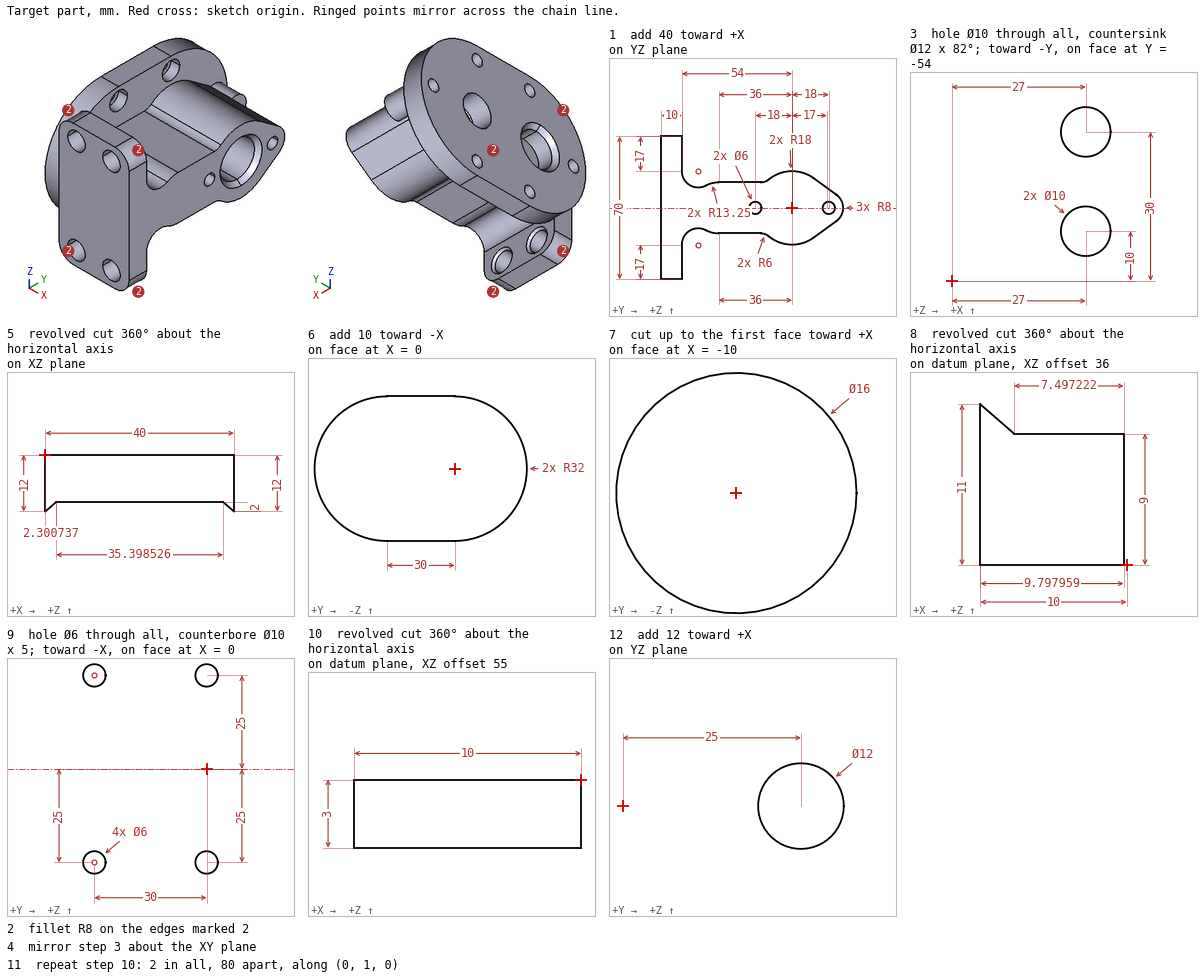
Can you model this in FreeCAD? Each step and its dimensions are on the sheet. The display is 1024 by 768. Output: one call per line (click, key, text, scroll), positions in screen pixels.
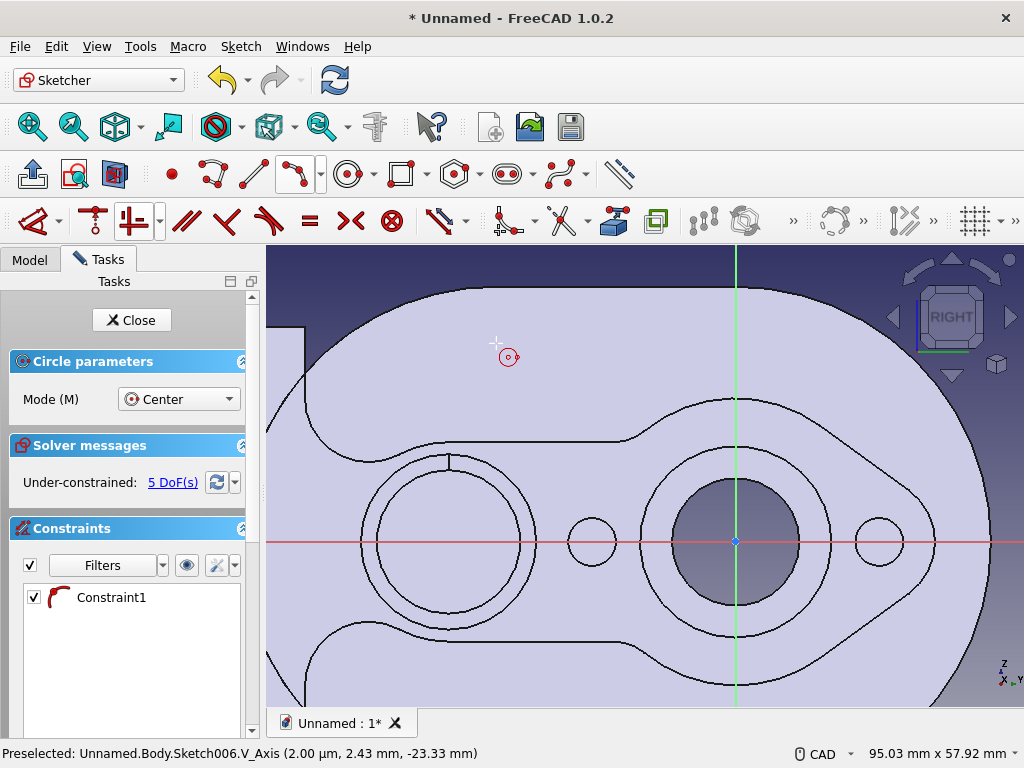
click(496, 343)
click(513, 326)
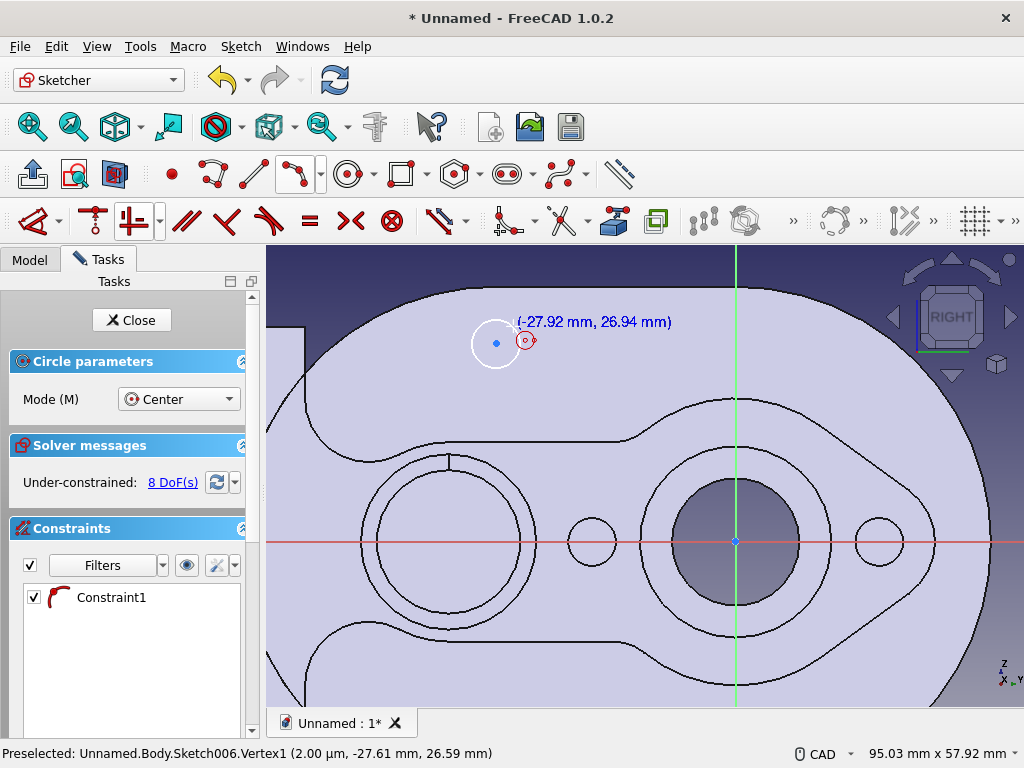
click(736, 343)
click(753, 326)
key(Escape)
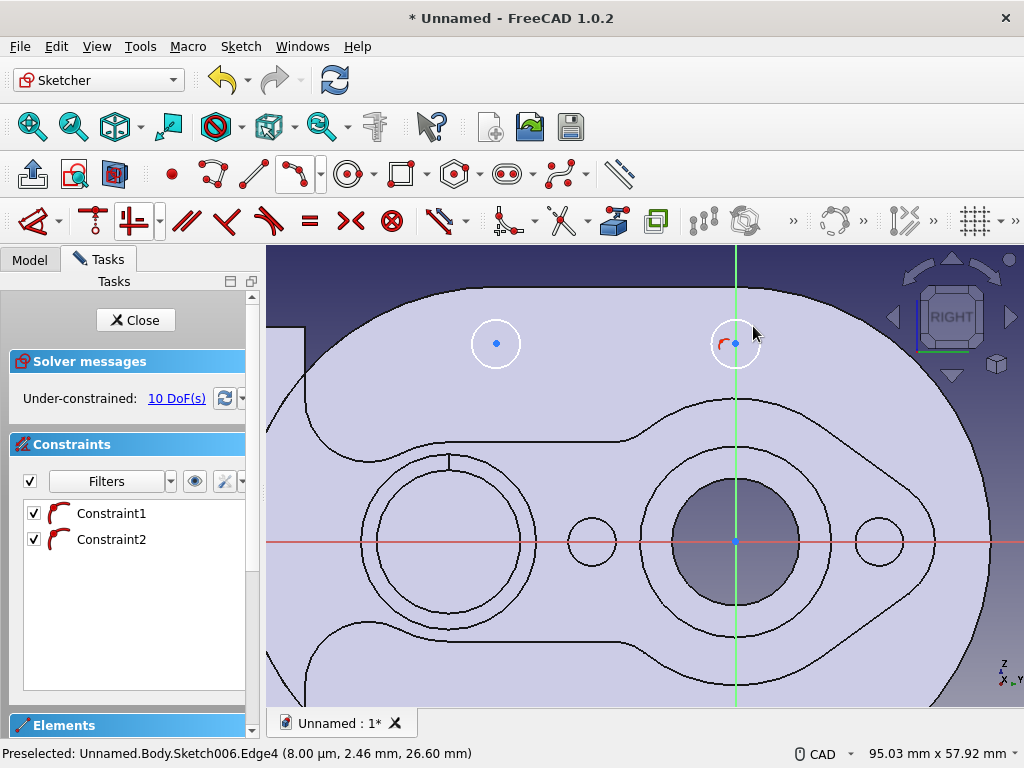
scroll(496, 342, down, 2)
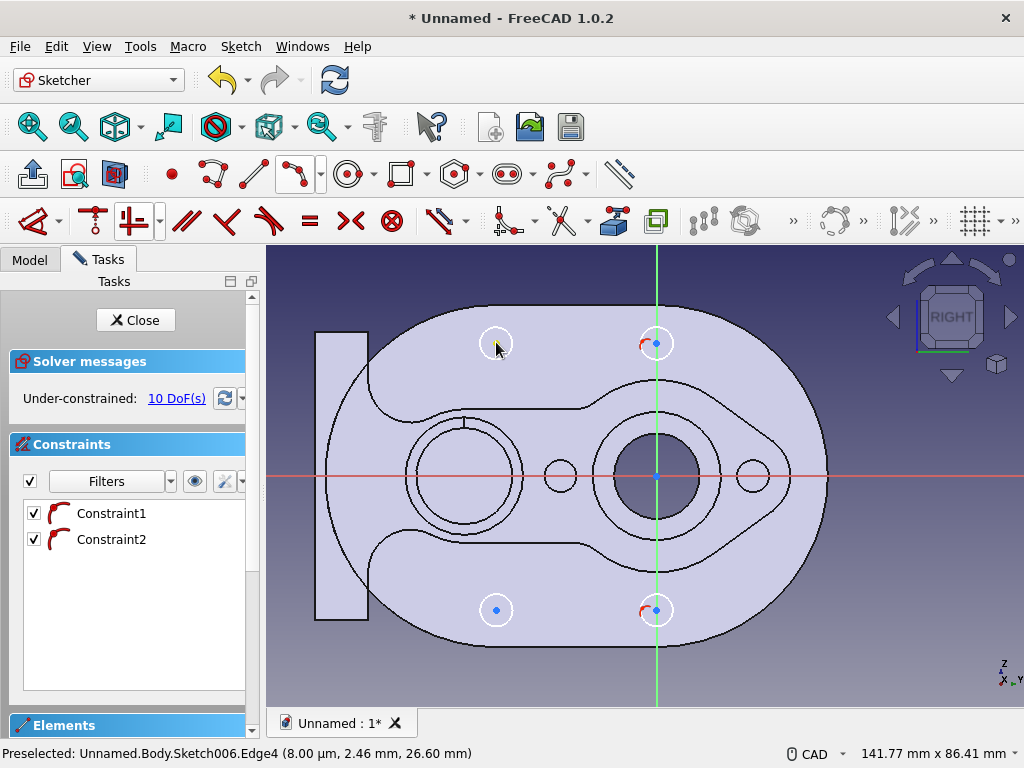
click(508, 599)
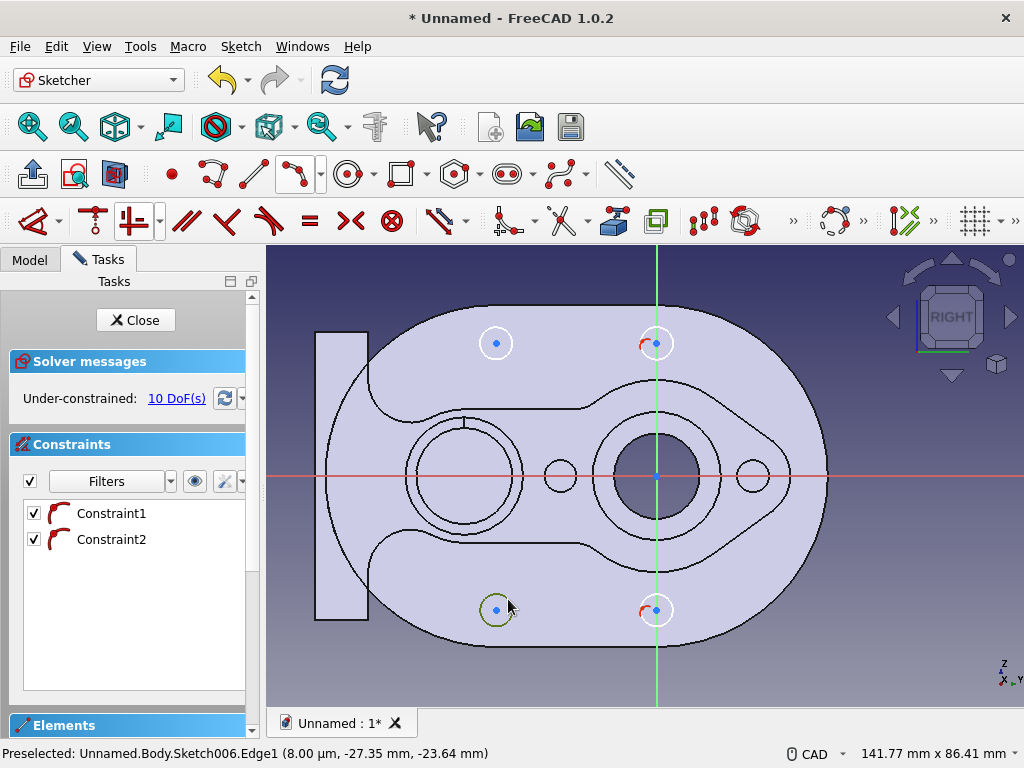
scroll(668, 599, up, 2)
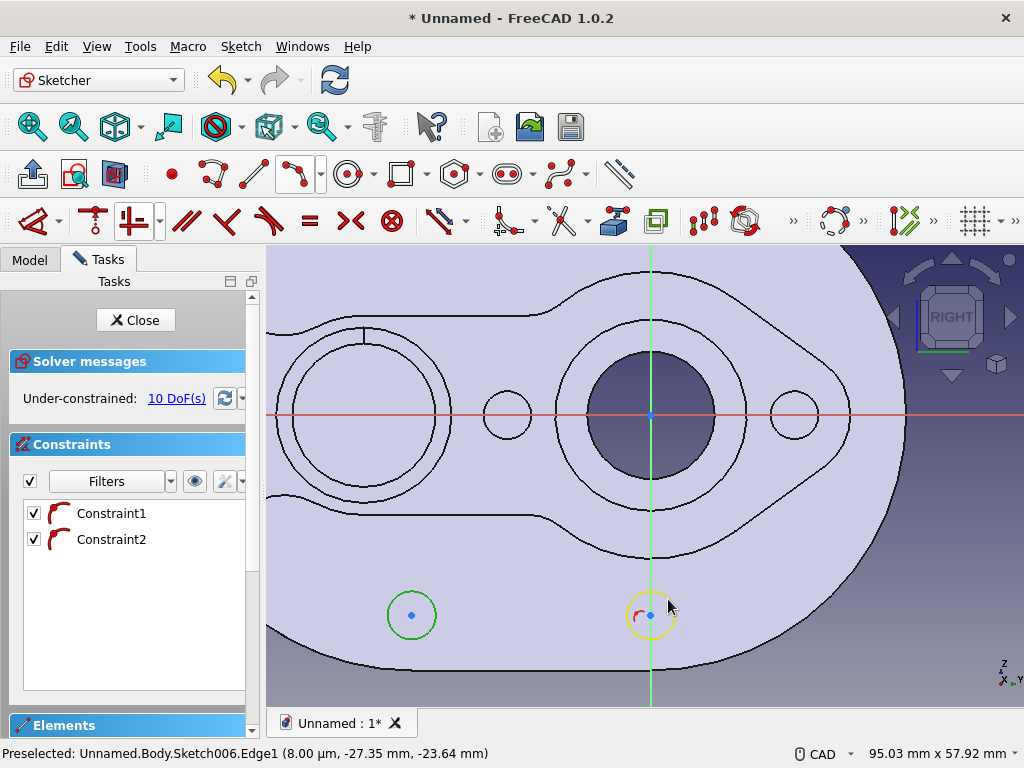
click(668, 598)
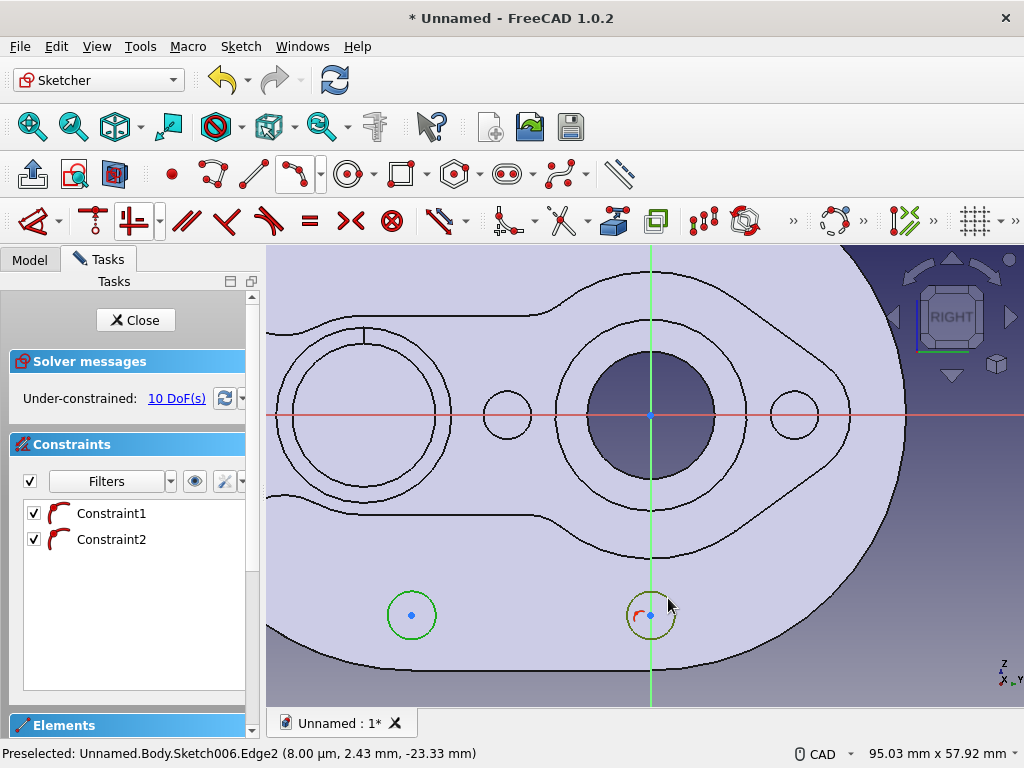
scroll(668, 600, down, 2)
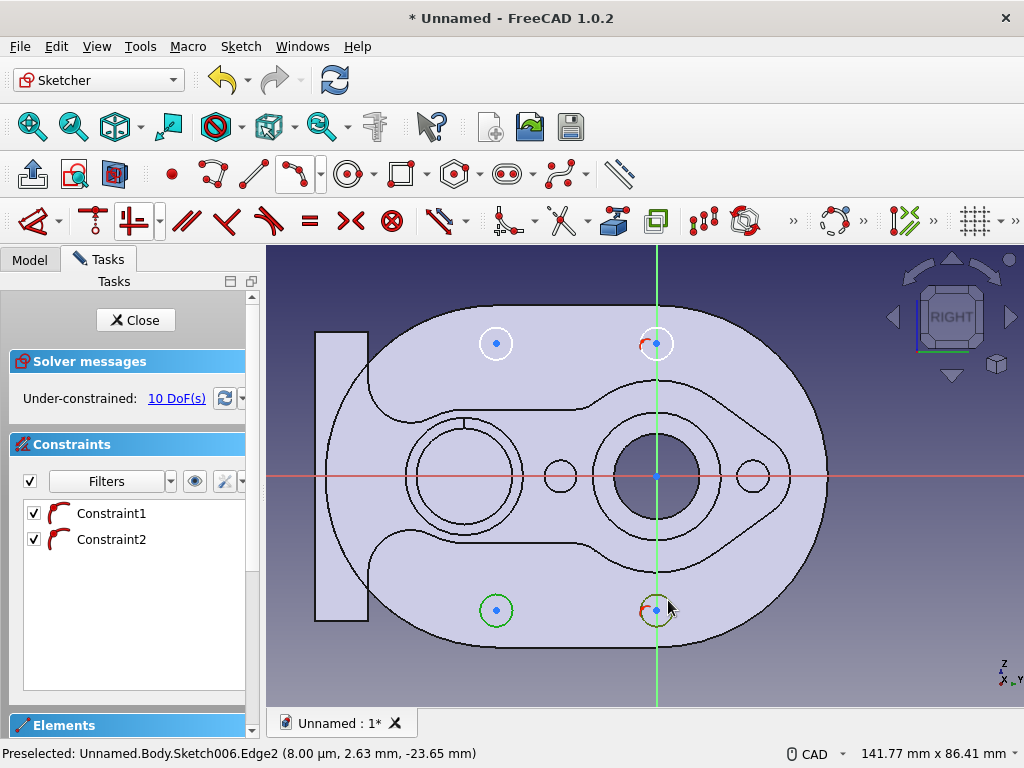
click(507, 332)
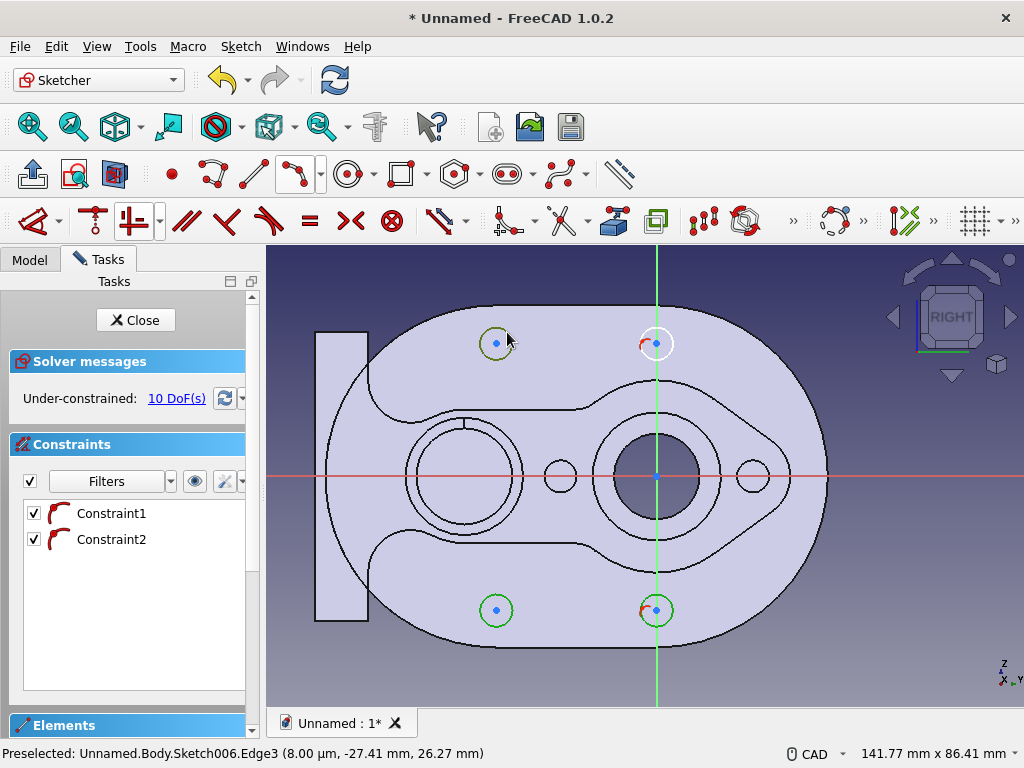
click(668, 332)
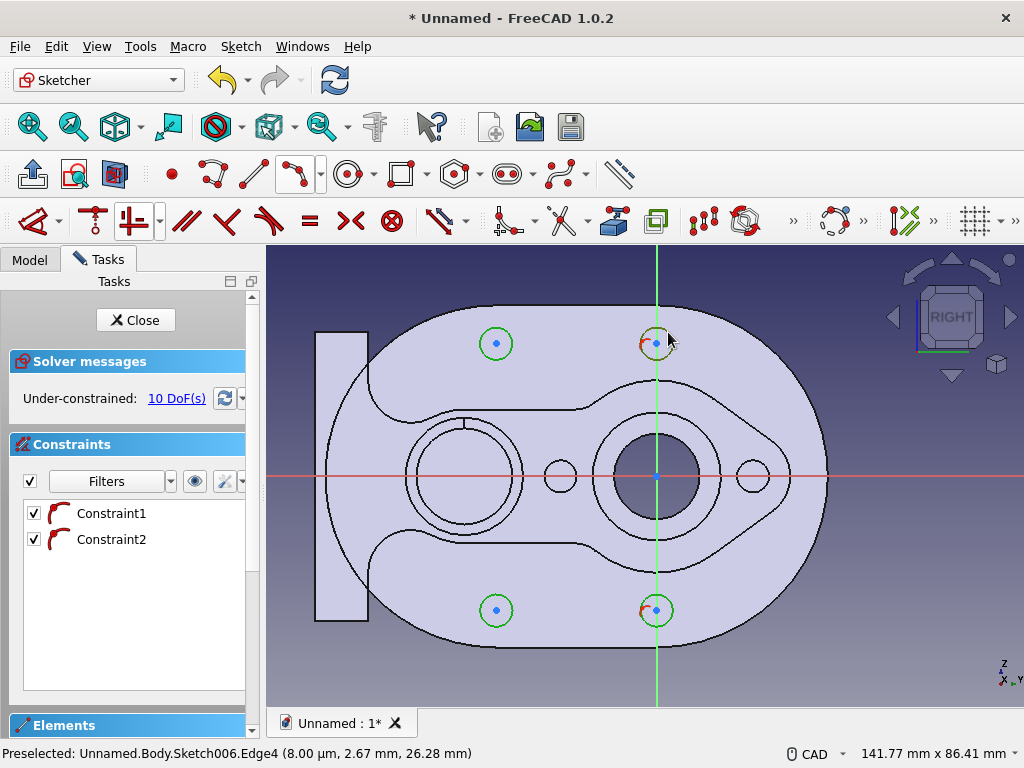
click(310, 222)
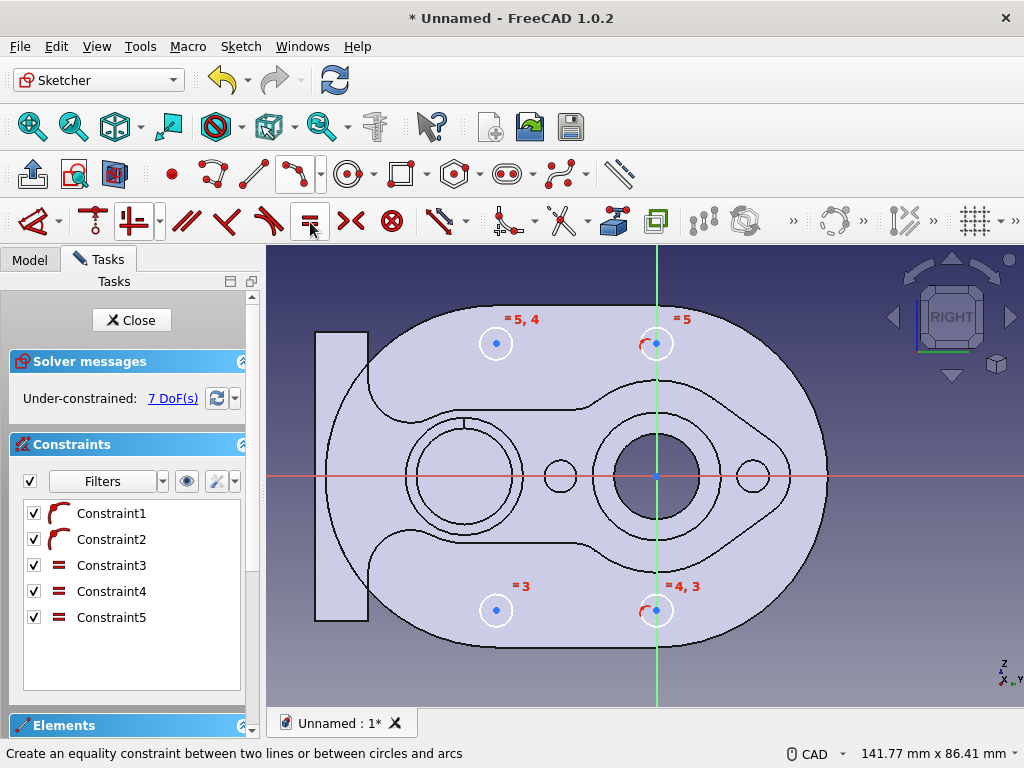
click(496, 611)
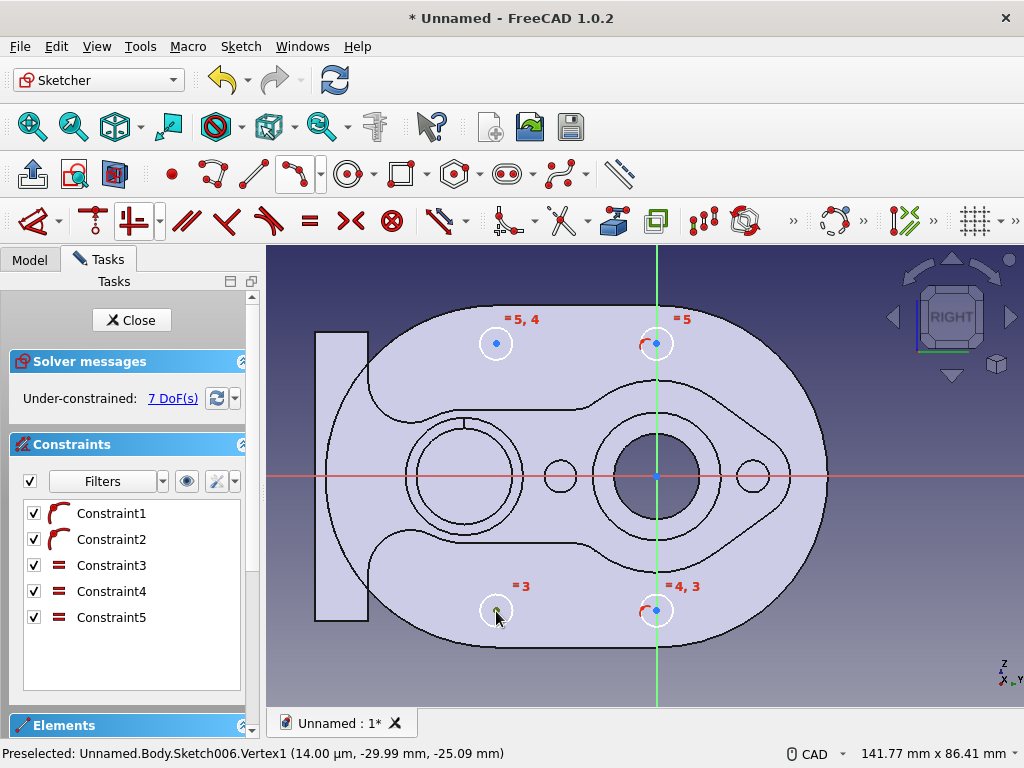
click(496, 344)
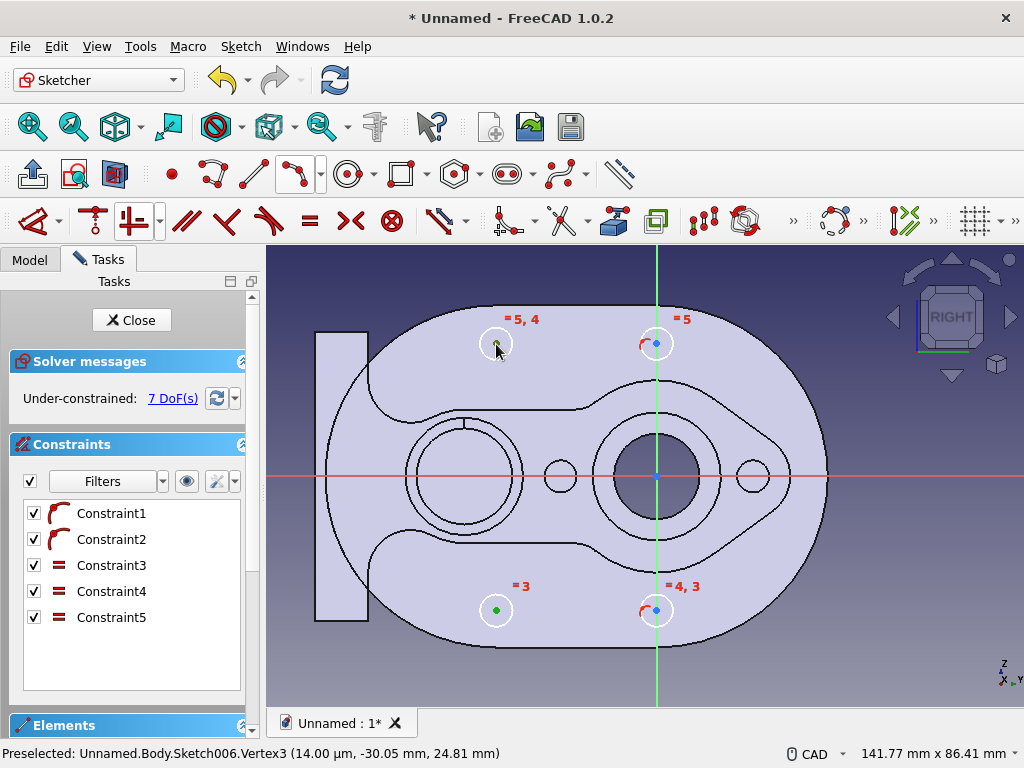
click(334, 476)